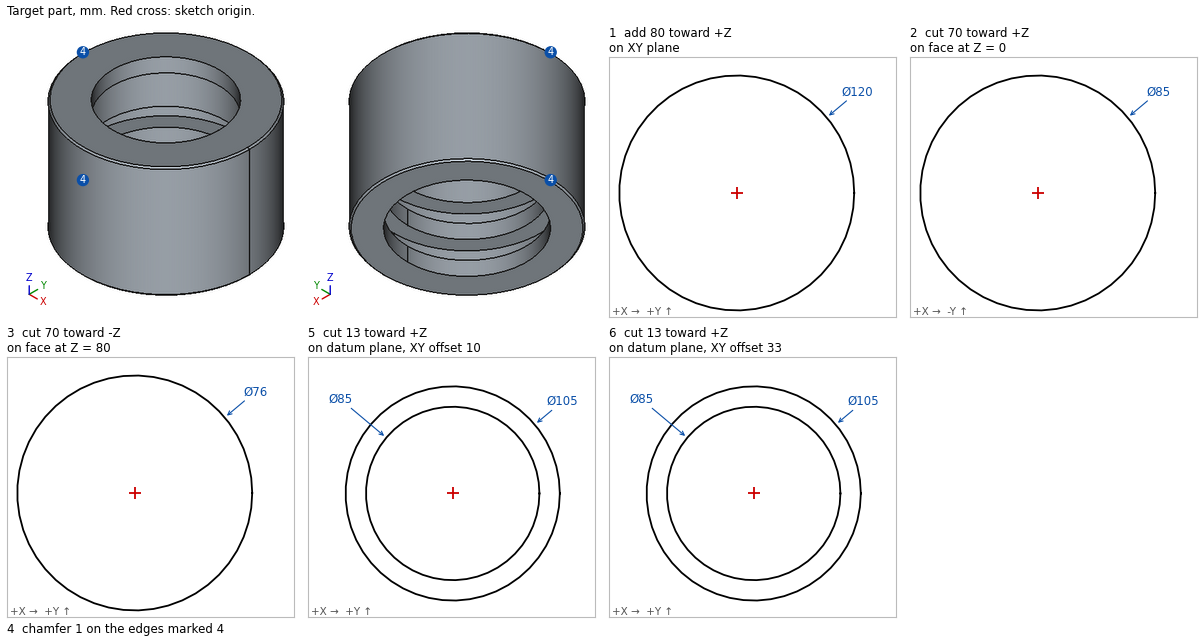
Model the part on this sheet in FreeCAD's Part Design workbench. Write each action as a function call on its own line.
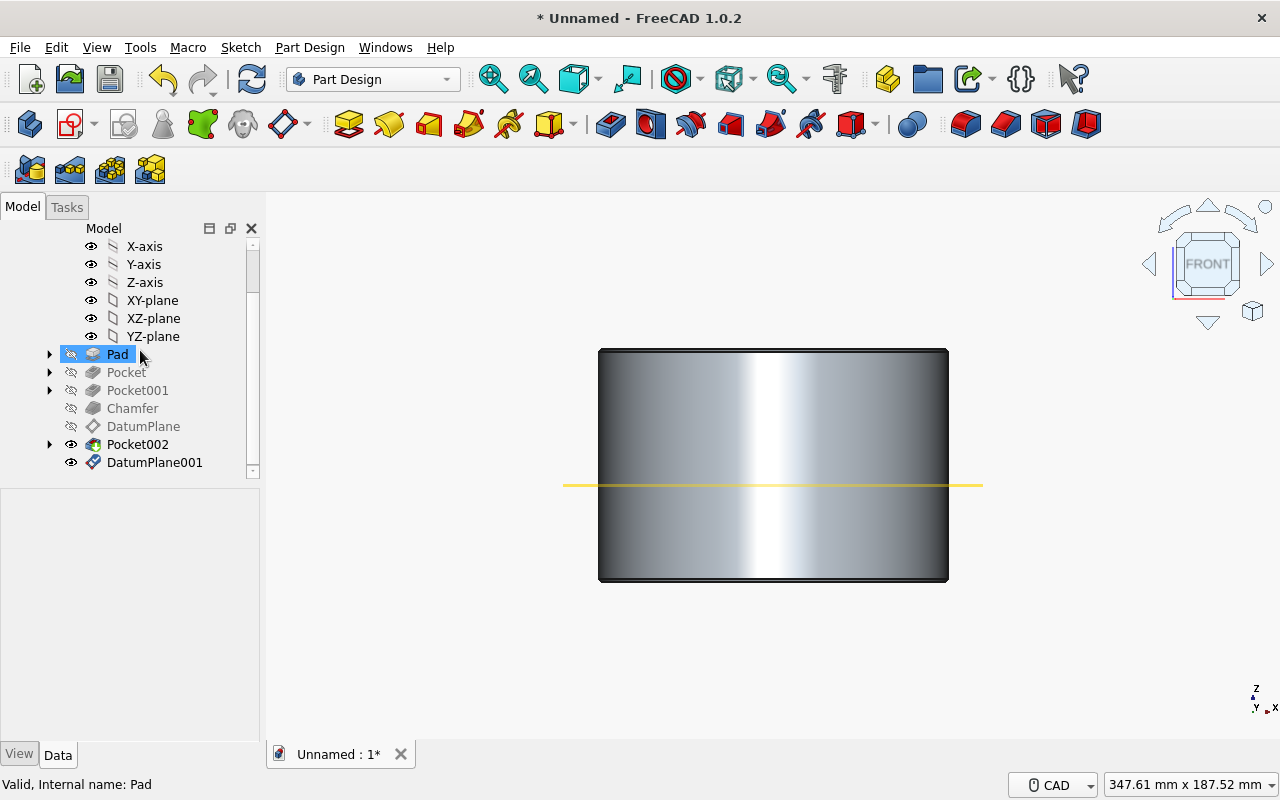
click(116, 462)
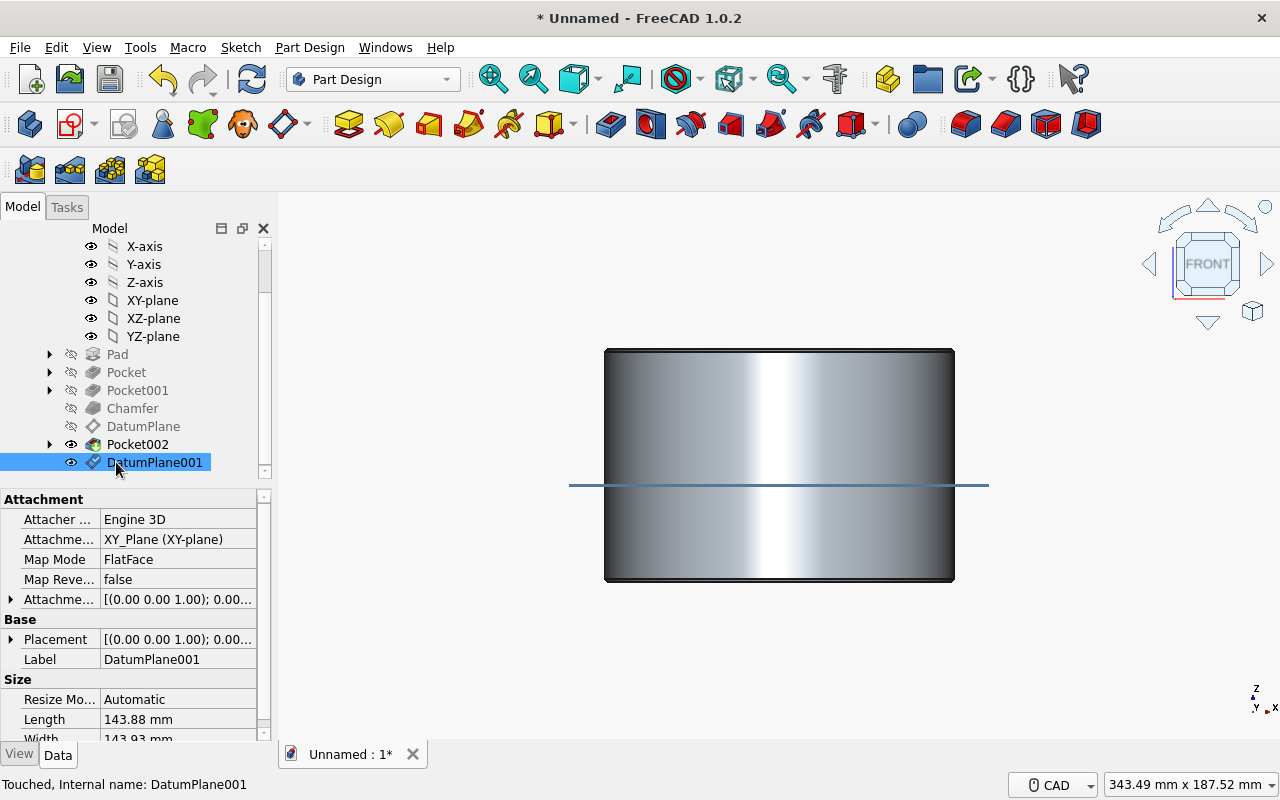
click(70, 124)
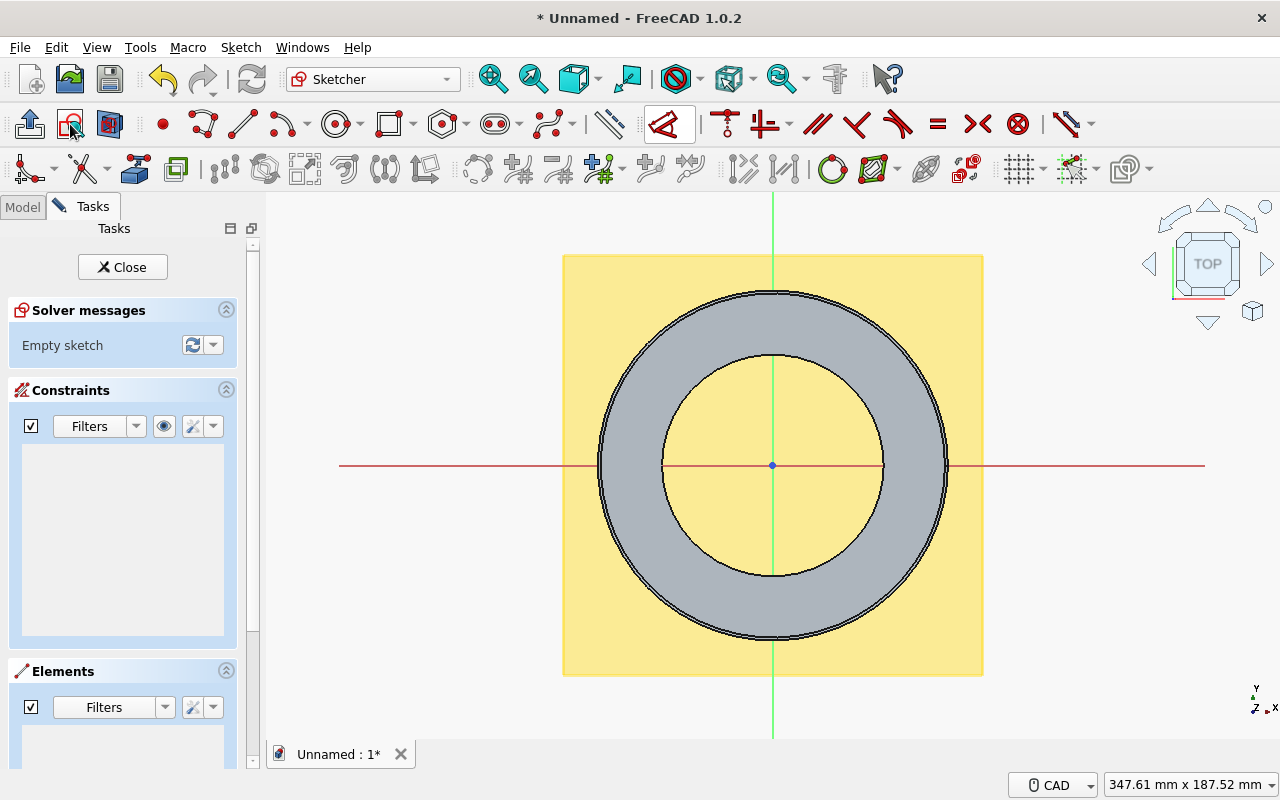
click(110, 124)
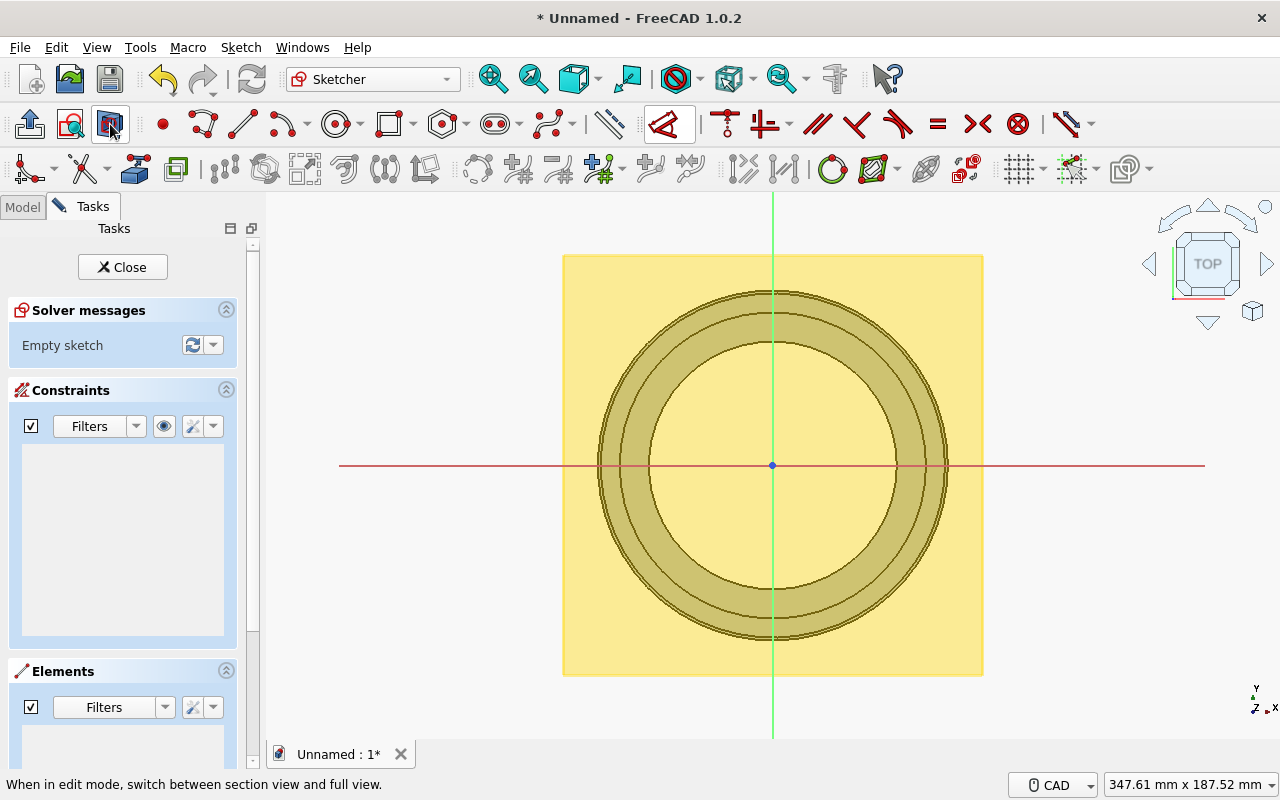
click(336, 124)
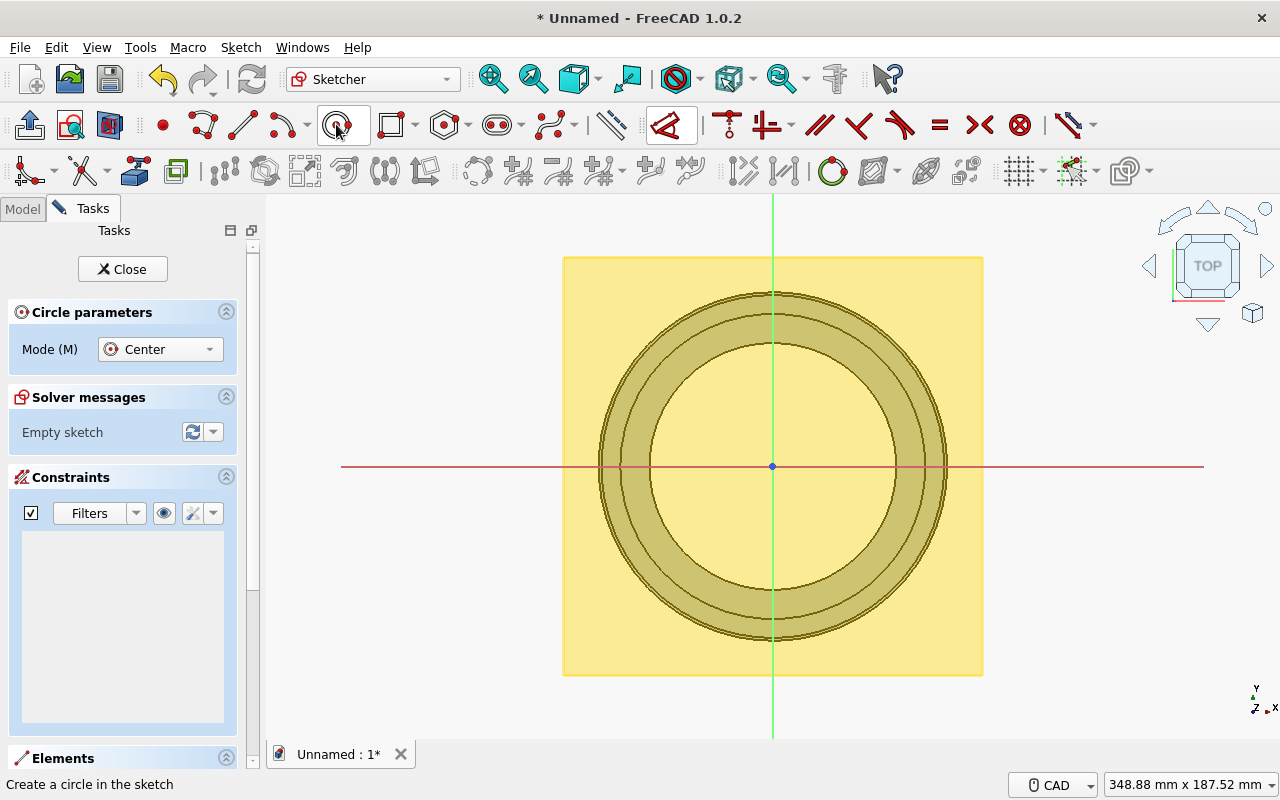
click(773, 466)
click(881, 359)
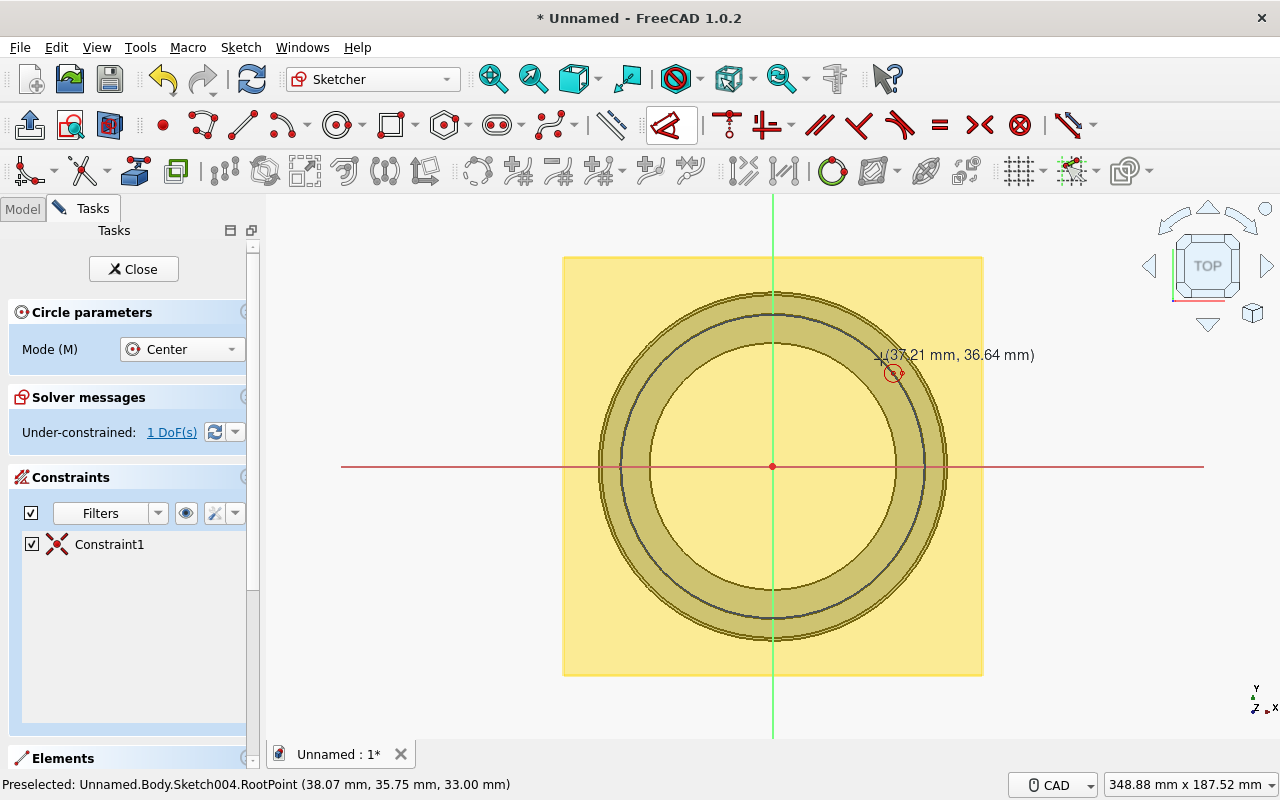
click(773, 466)
click(860, 379)
key(Escape)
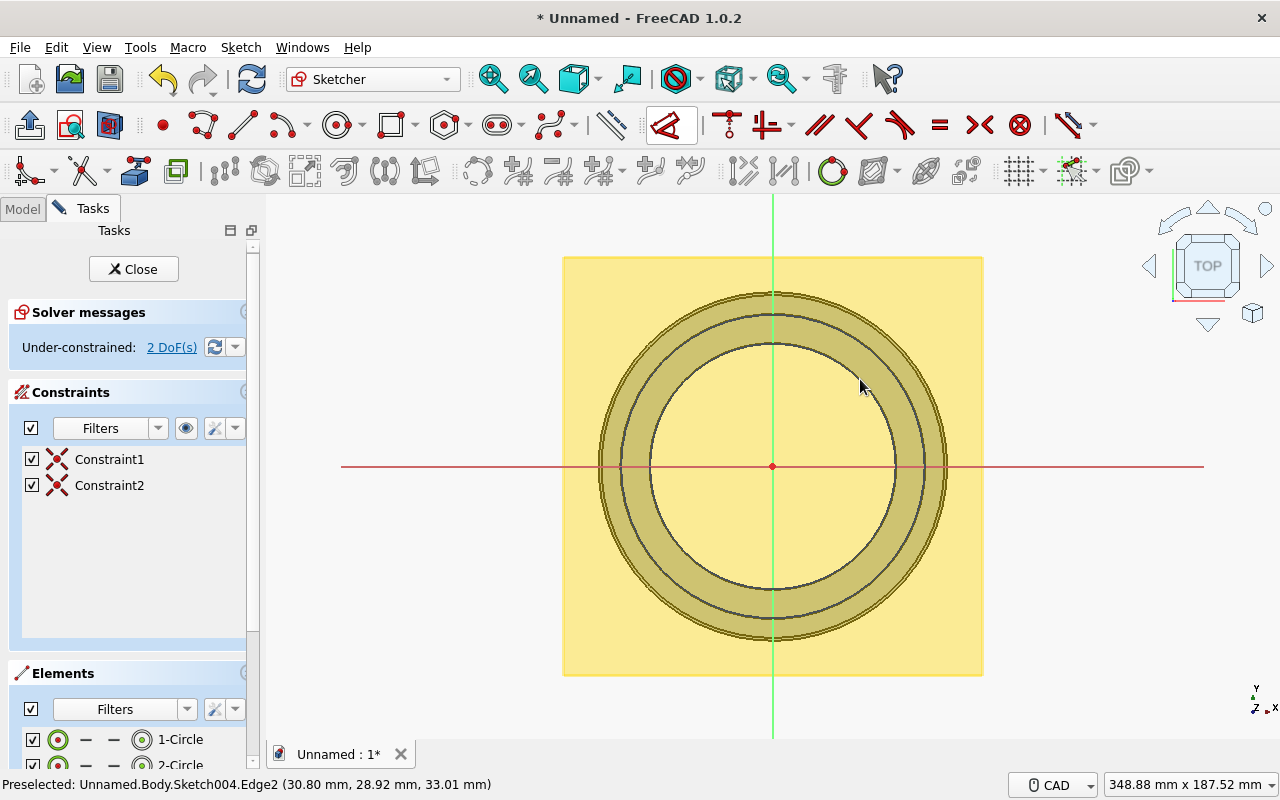
click(880, 359)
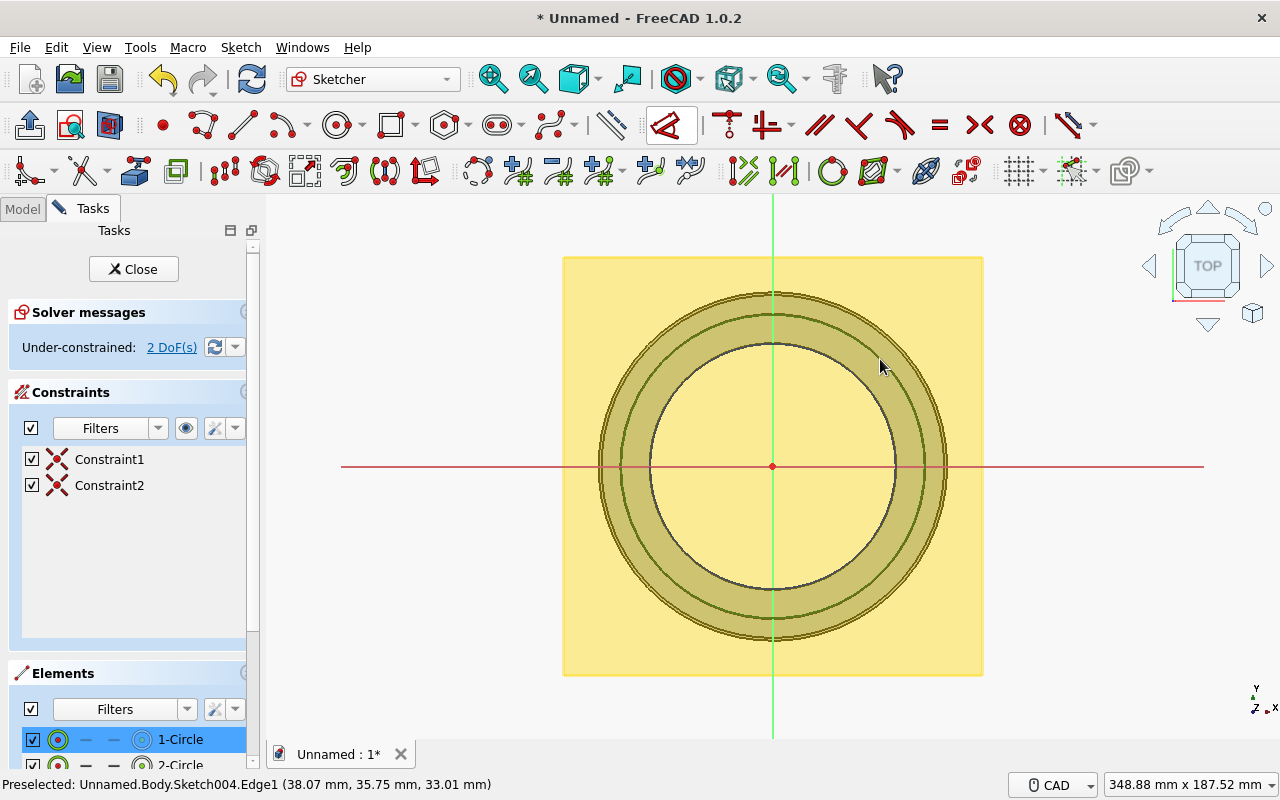
click(692, 126)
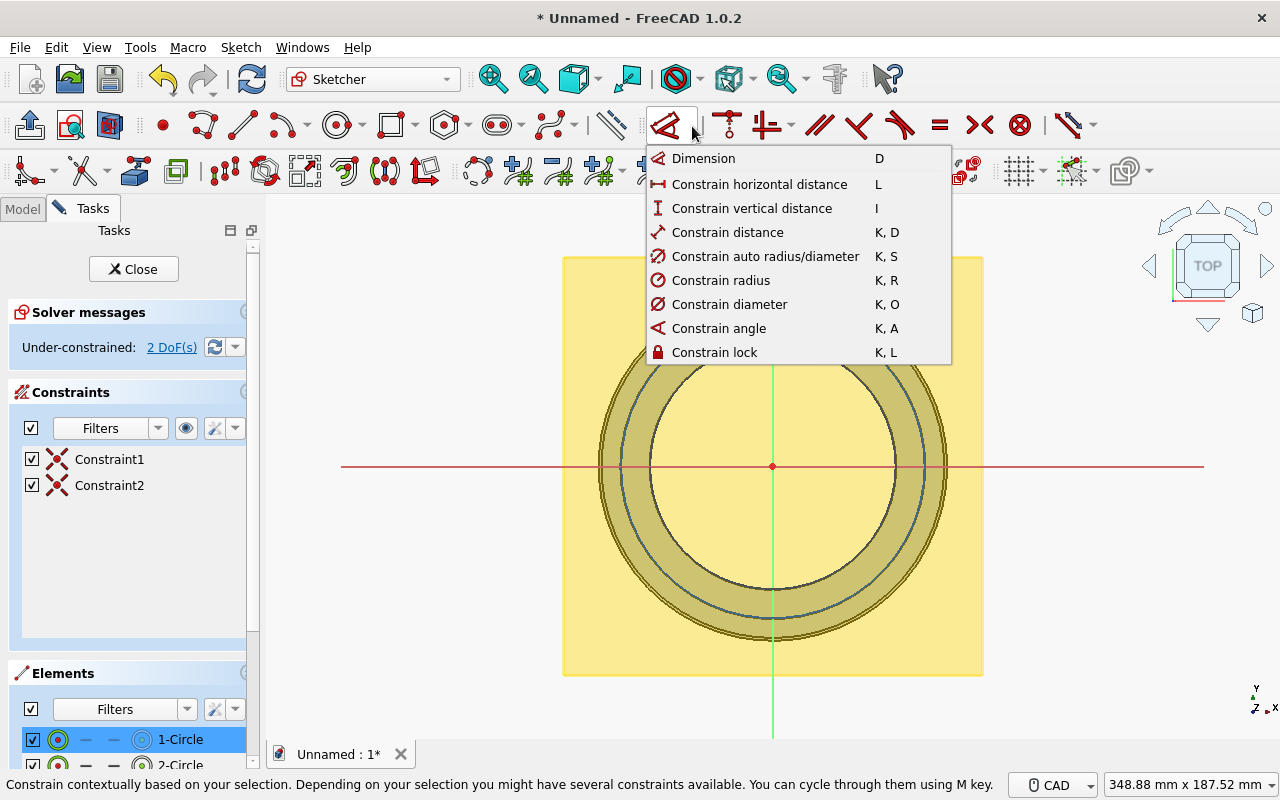
click(799, 304)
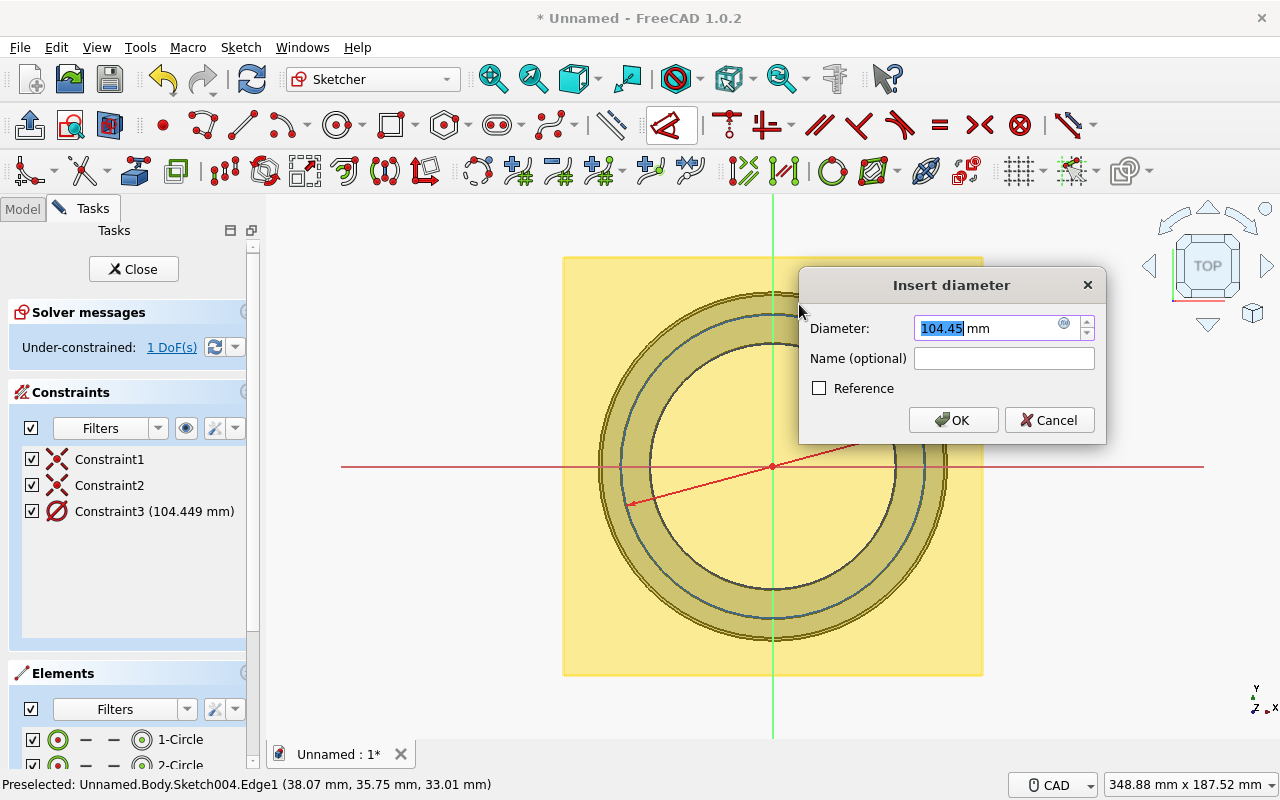
text(105)
key(Return)